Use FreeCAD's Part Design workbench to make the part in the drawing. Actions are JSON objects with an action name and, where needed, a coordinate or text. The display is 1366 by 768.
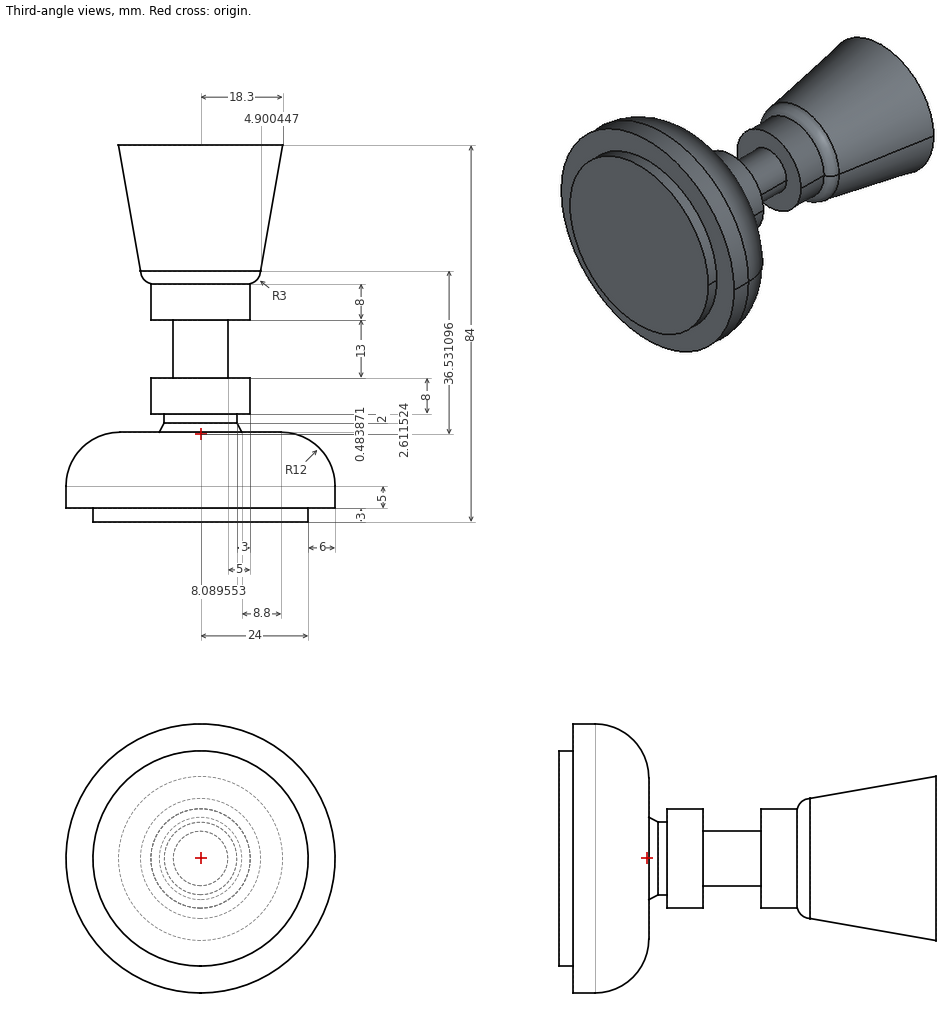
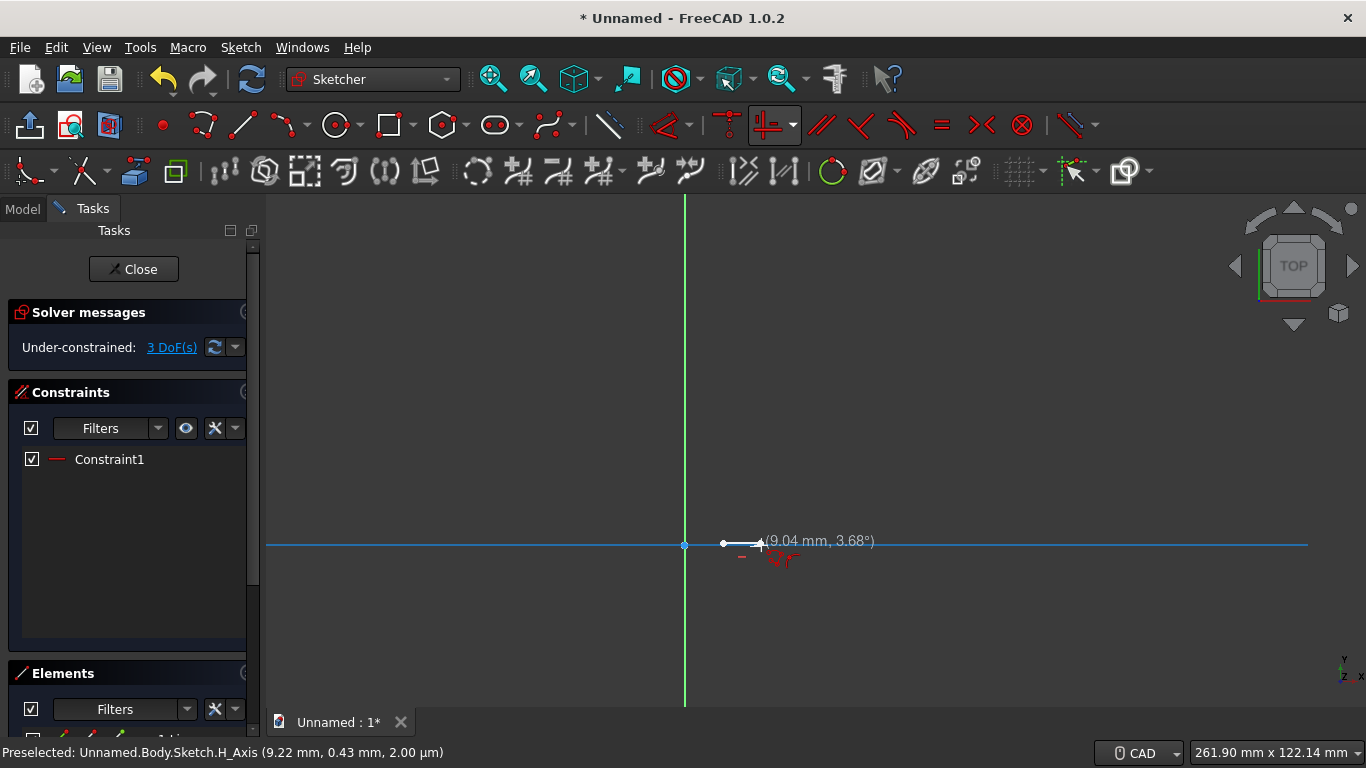
{"action": "scroll", "coordinate": [719, 534], "scroll_direction": "up", "scroll_amount": 3}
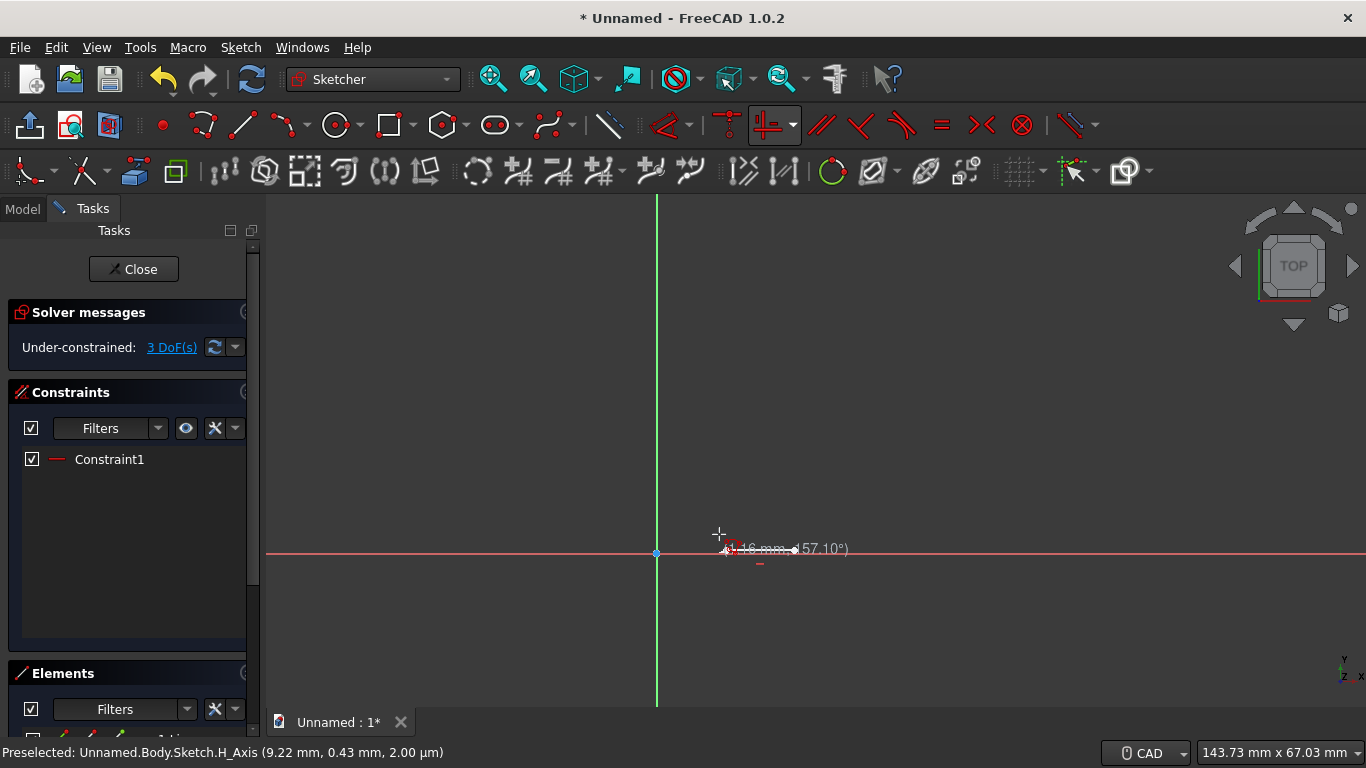
{"action": "left_click", "coordinate": [718, 534]}
{"action": "left_click", "coordinate": [718, 519]}
{"action": "left_click", "coordinate": [741, 519]}
{"action": "left_click", "coordinate": [741, 457]}
{"action": "left_click", "coordinate": [703, 457]}
{"action": "left_click", "coordinate": [703, 358]}
{"action": "left_click", "coordinate": [741, 358]}
{"action": "left_click", "coordinate": [741, 297]}
{"action": "right_click", "coordinate": [741, 297]}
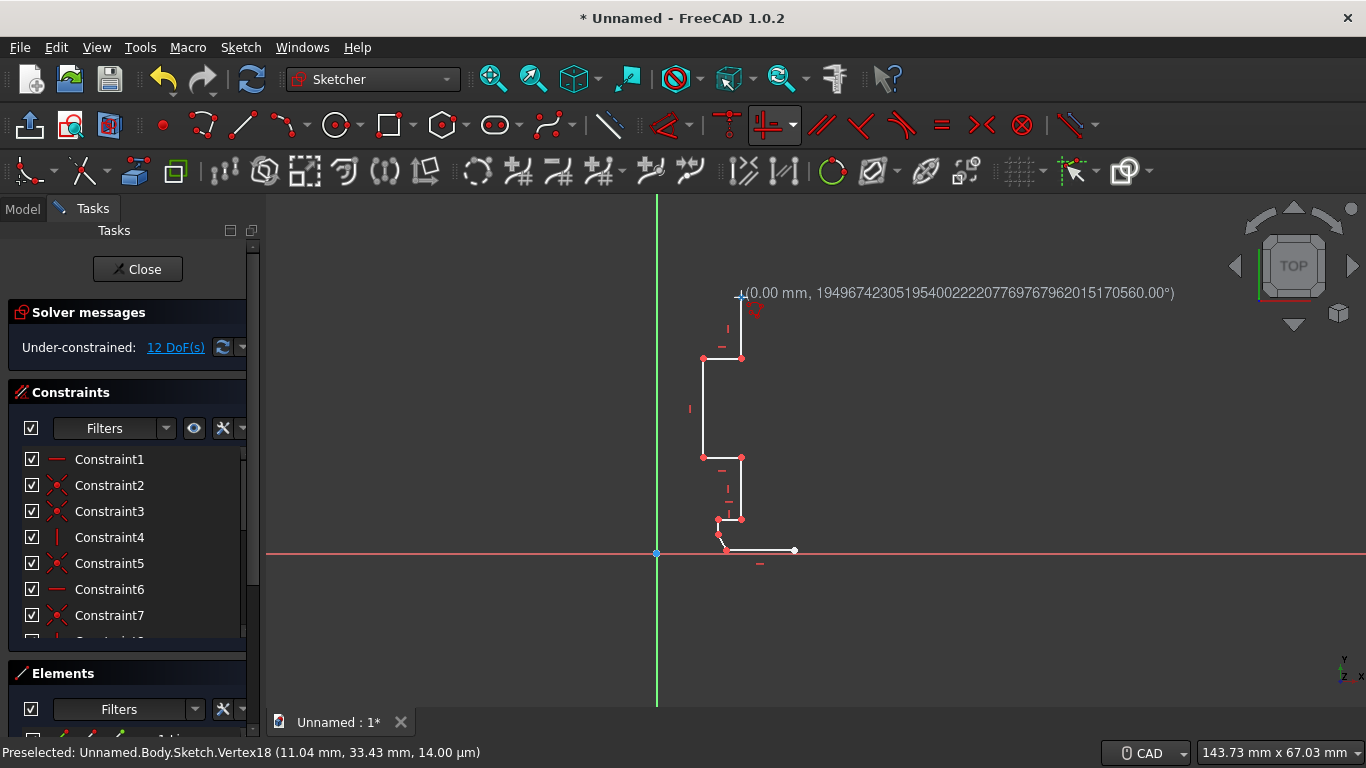
{"action": "left_click", "coordinate": [759, 274]}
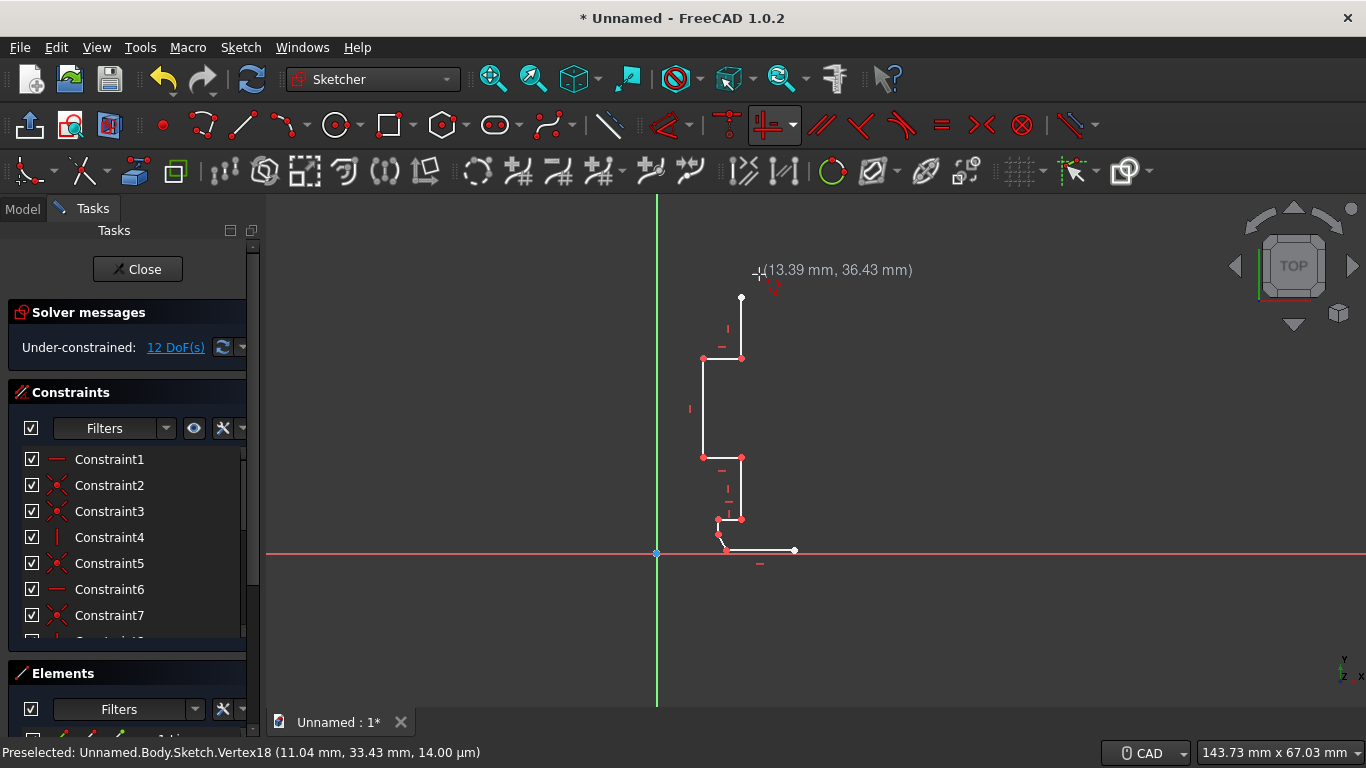
{"action": "scroll", "coordinate": [719, 534], "scroll_direction": "down", "scroll_amount": 3}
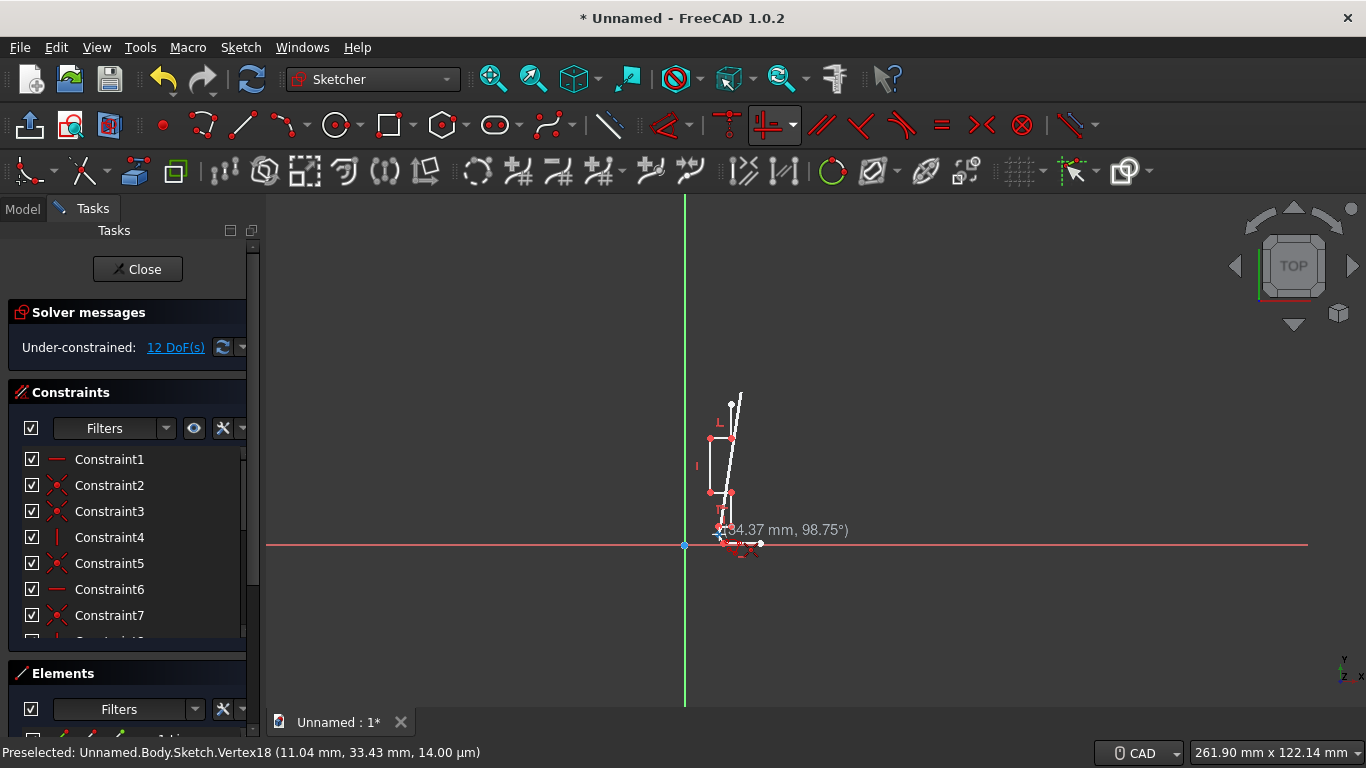
{"action": "left_click", "coordinate": [762, 274]}
{"action": "left_click", "coordinate": [685, 274]}
{"action": "left_click", "coordinate": [694, 627]}
{"action": "left_click", "coordinate": [786, 627]}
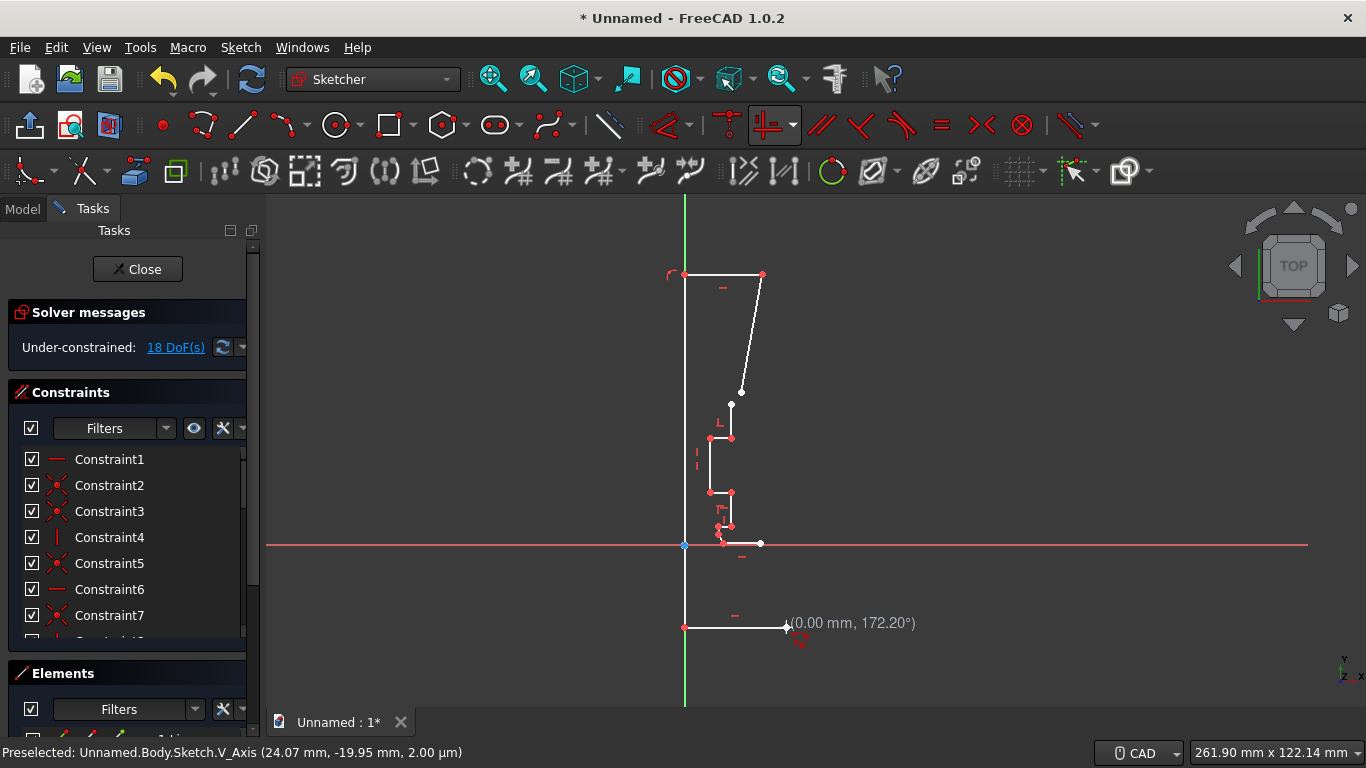
{"action": "scroll", "coordinate": [786, 615], "scroll_direction": "up", "scroll_amount": 2}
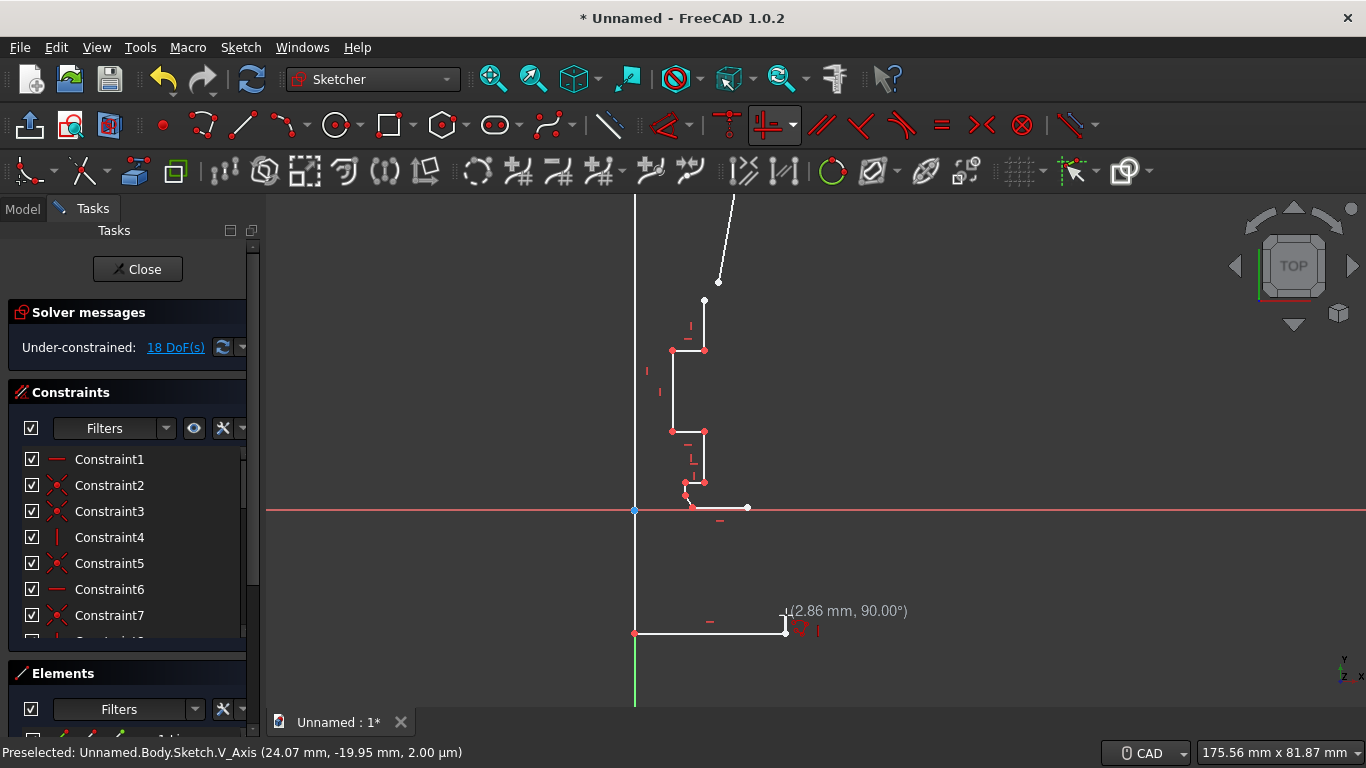
{"action": "left_click", "coordinate": [786, 614]}
{"action": "left_click", "coordinate": [823, 614]}
{"action": "left_click", "coordinate": [823, 583]}
{"action": "right_click", "coordinate": [823, 583]}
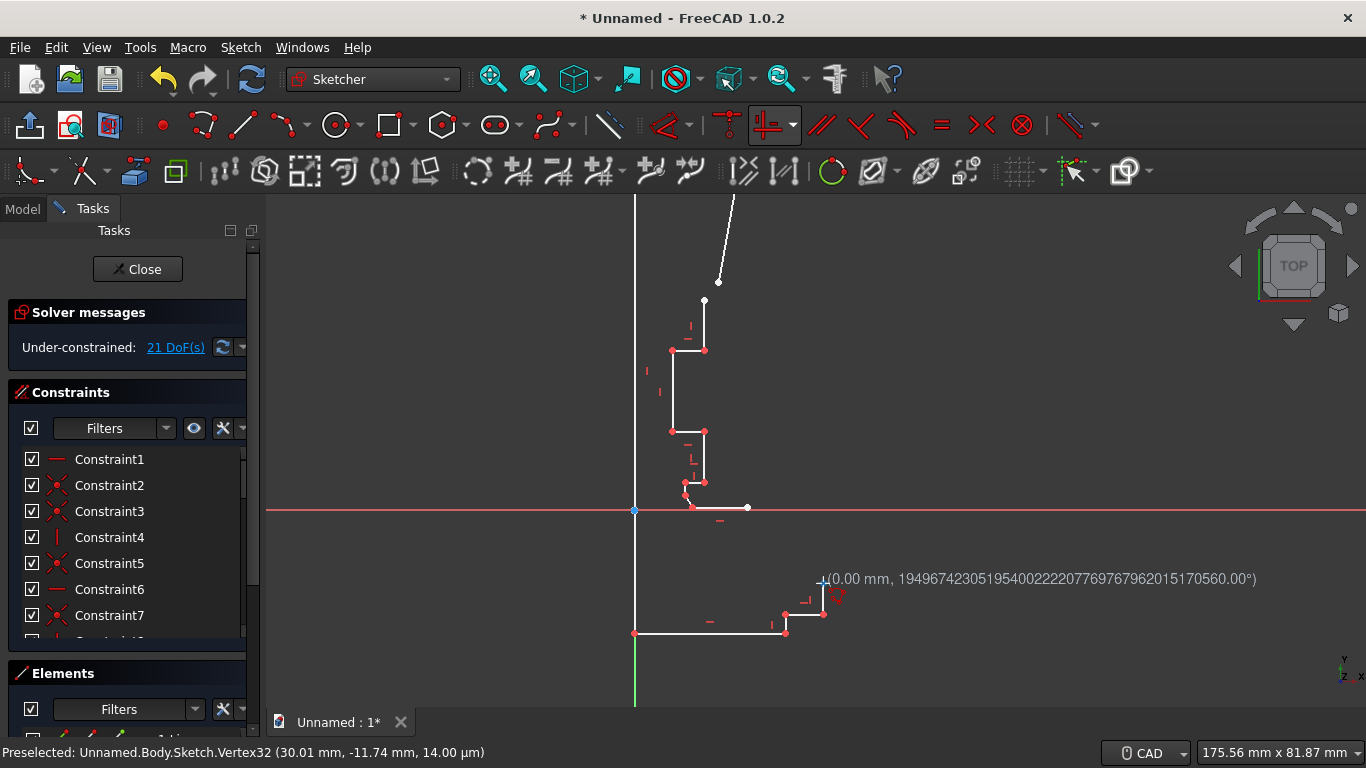
{"action": "key", "text": "g 3 a"}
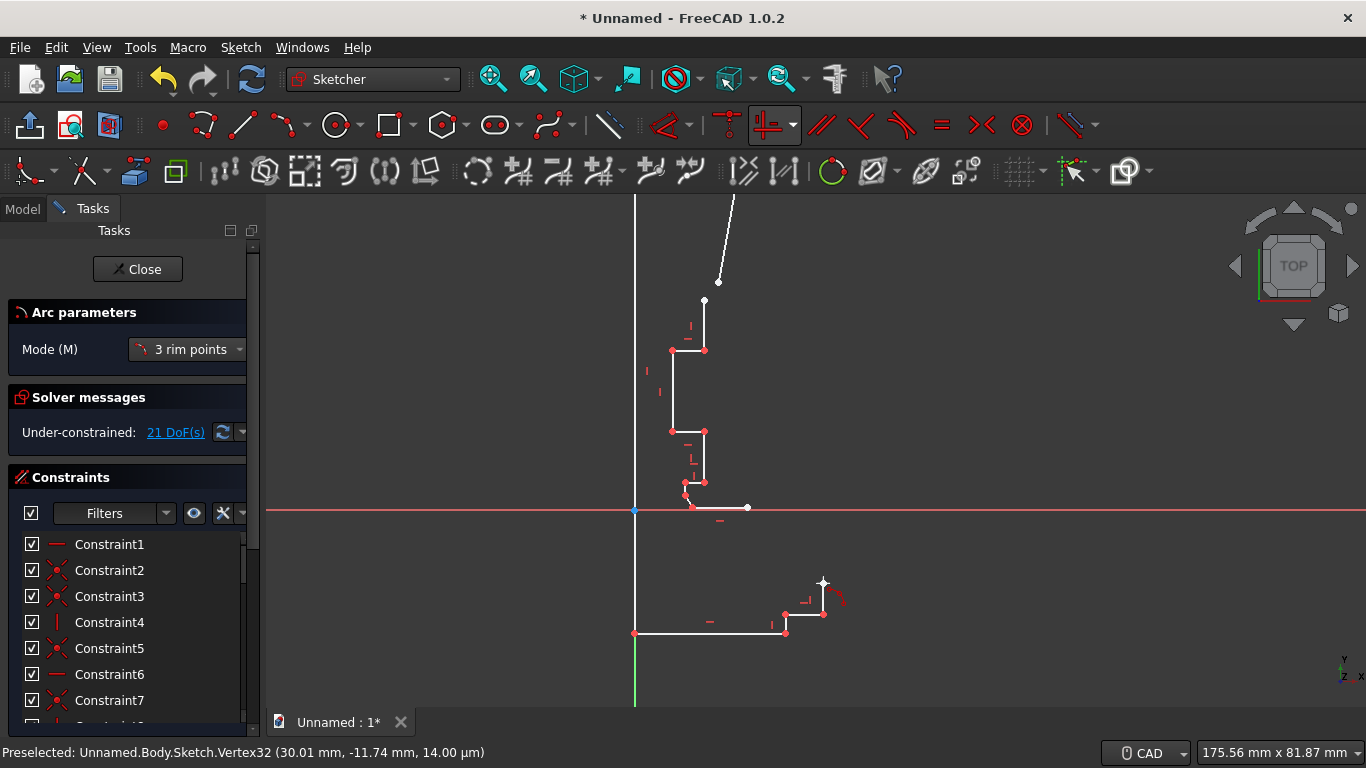
{"action": "left_click", "coordinate": [704, 301]}
{"action": "left_click", "coordinate": [719, 282]}